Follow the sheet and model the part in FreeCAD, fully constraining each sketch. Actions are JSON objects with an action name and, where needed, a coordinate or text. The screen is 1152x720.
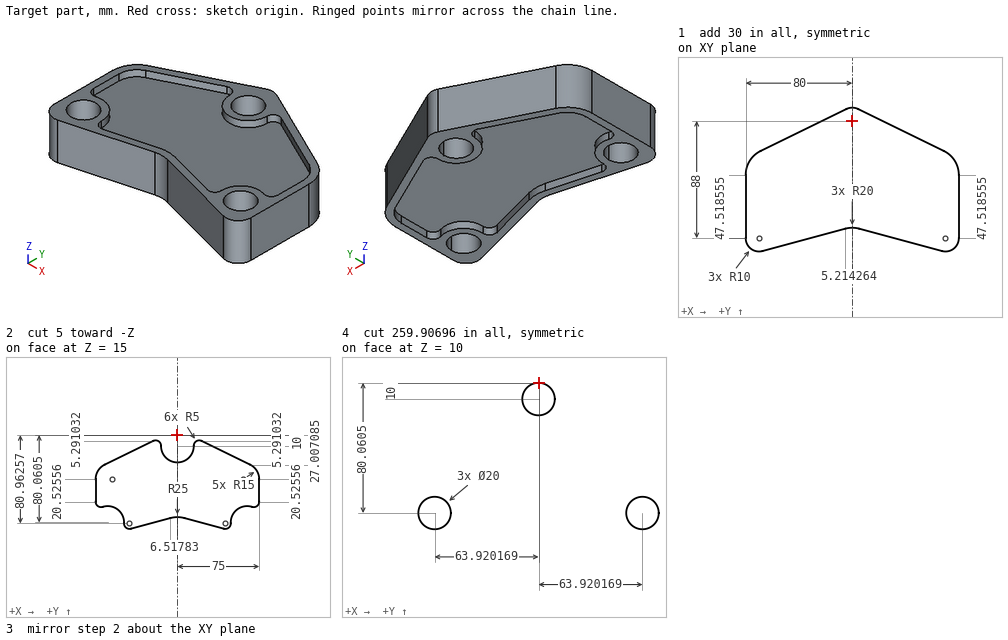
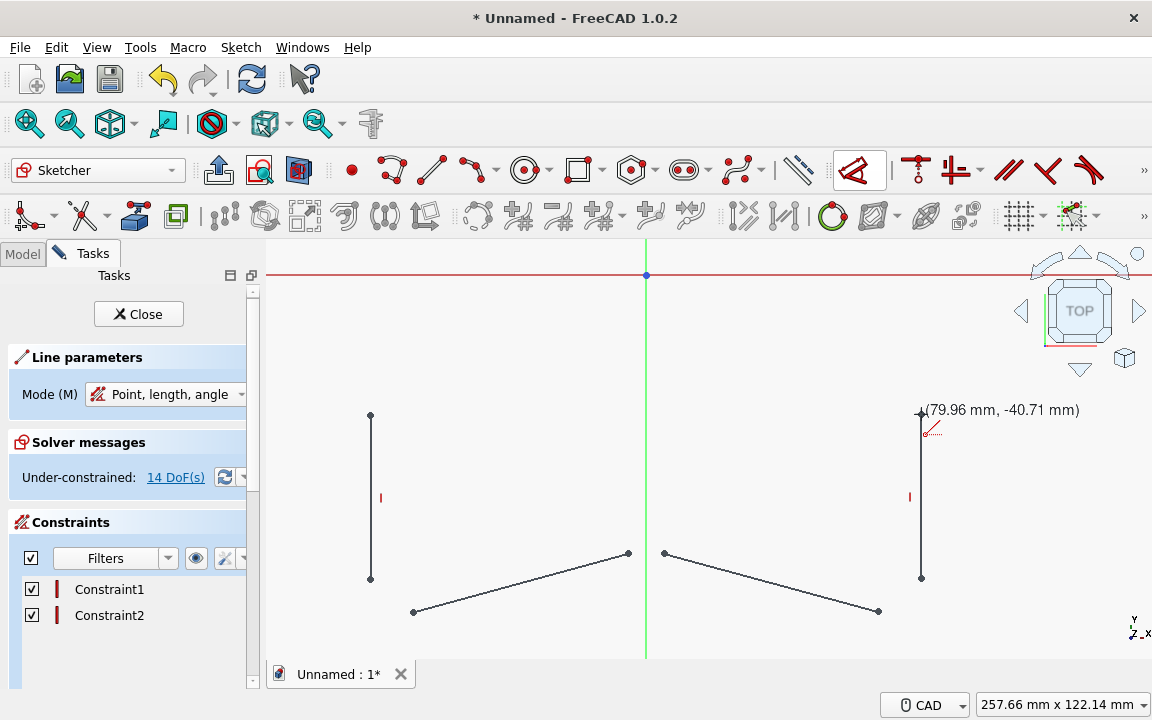
{"action": "left_click", "coordinate": [883, 352]}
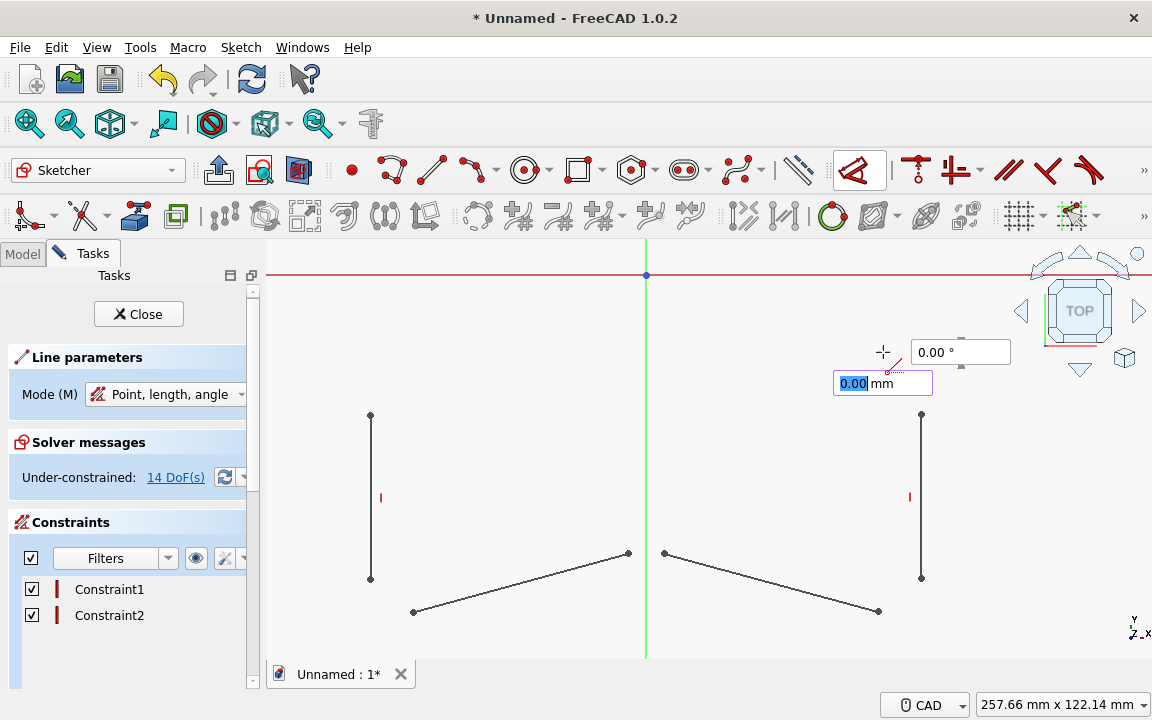
{"action": "scroll", "coordinate": [629, 496], "scroll_direction": "down", "scroll_amount": 2}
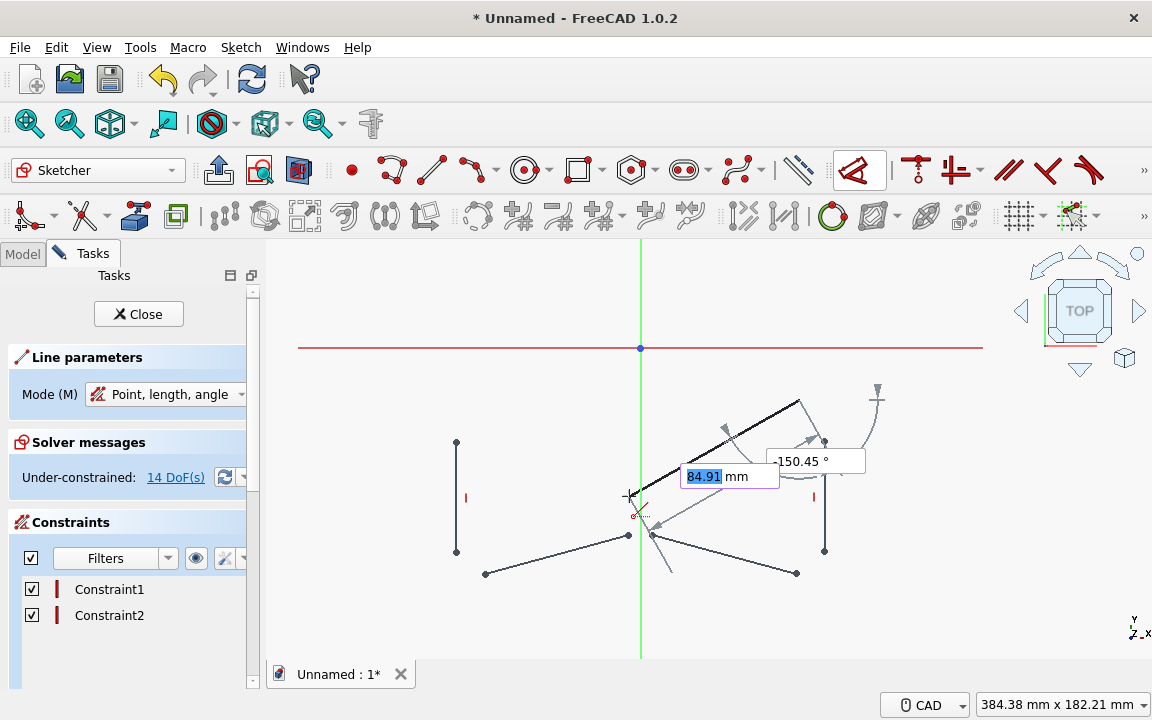
{"action": "scroll", "coordinate": [651, 327], "scroll_direction": "up", "scroll_amount": 3}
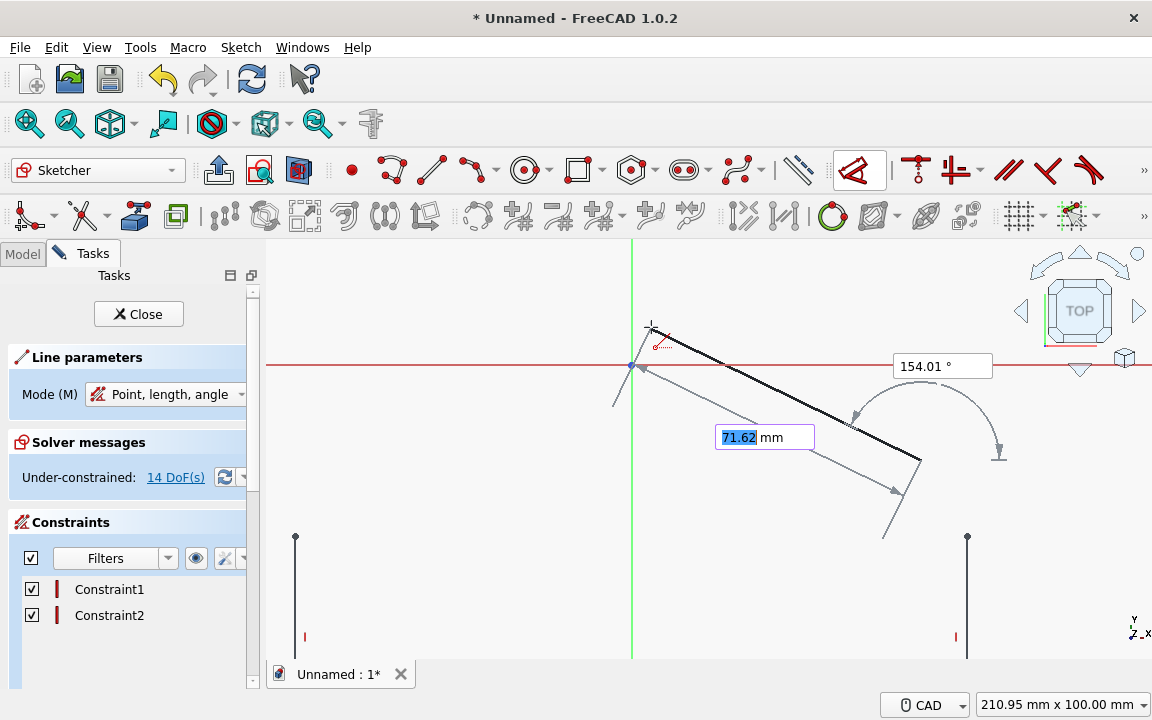
{"action": "left_click", "coordinate": [650, 328]}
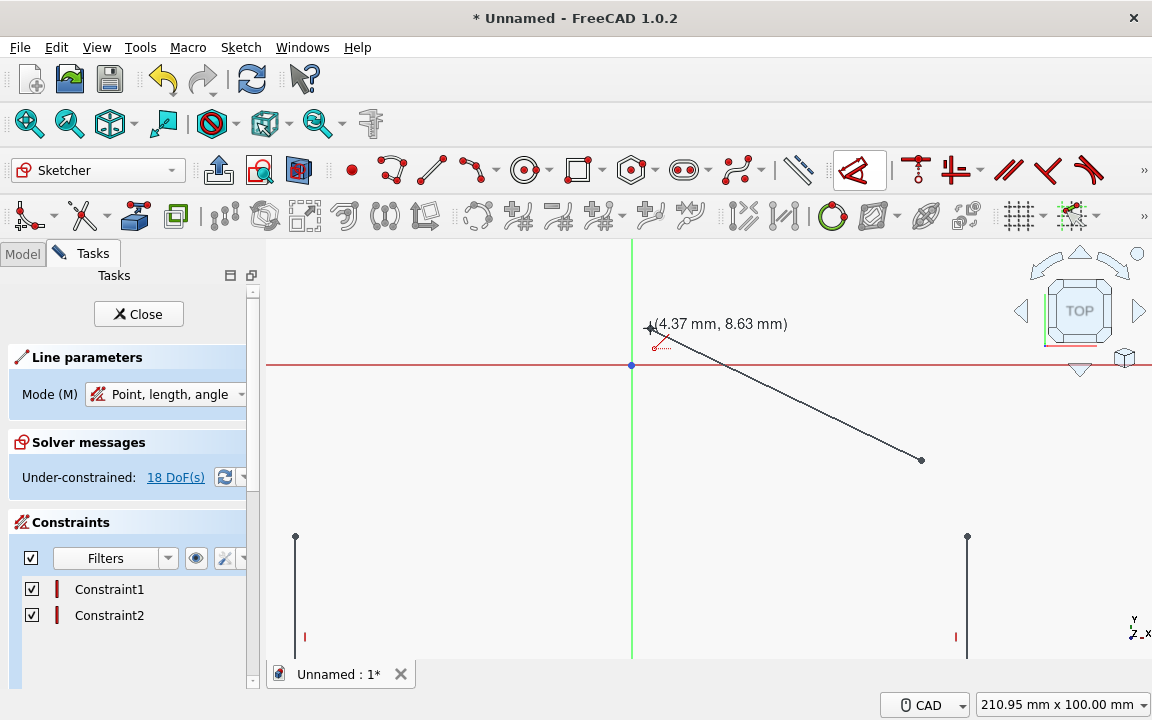
{"action": "left_click", "coordinate": [613, 328]}
{"action": "left_click", "coordinate": [343, 460]}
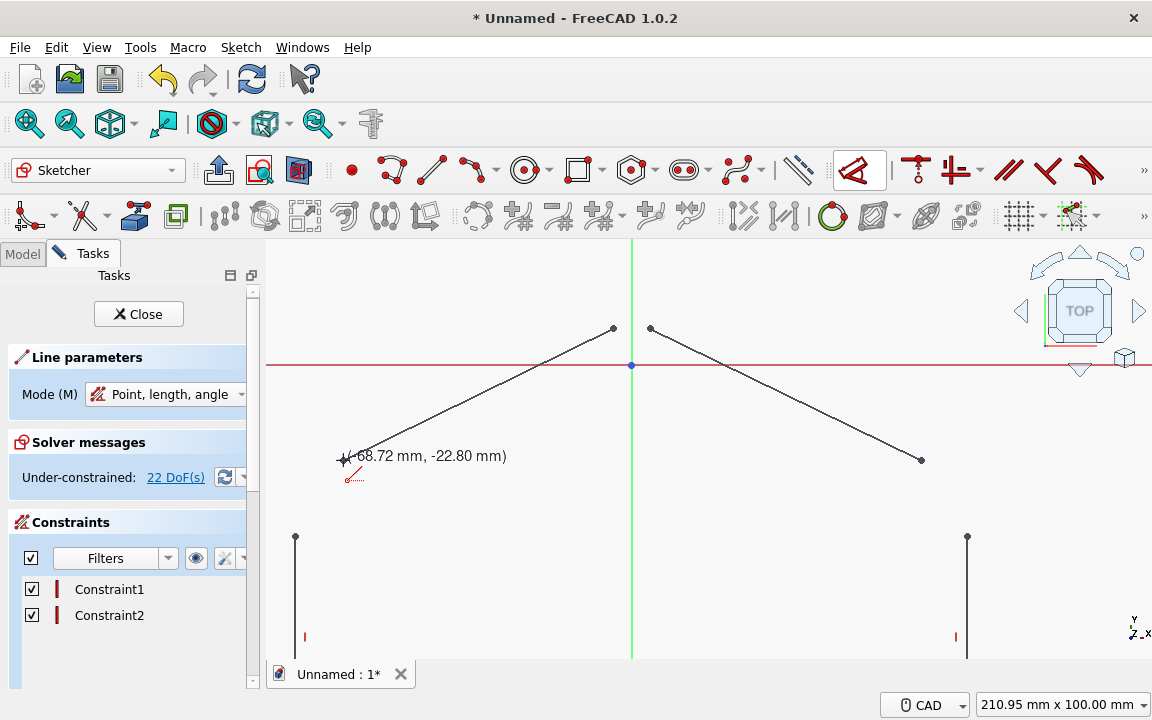
{"action": "left_click", "coordinate": [472, 170]}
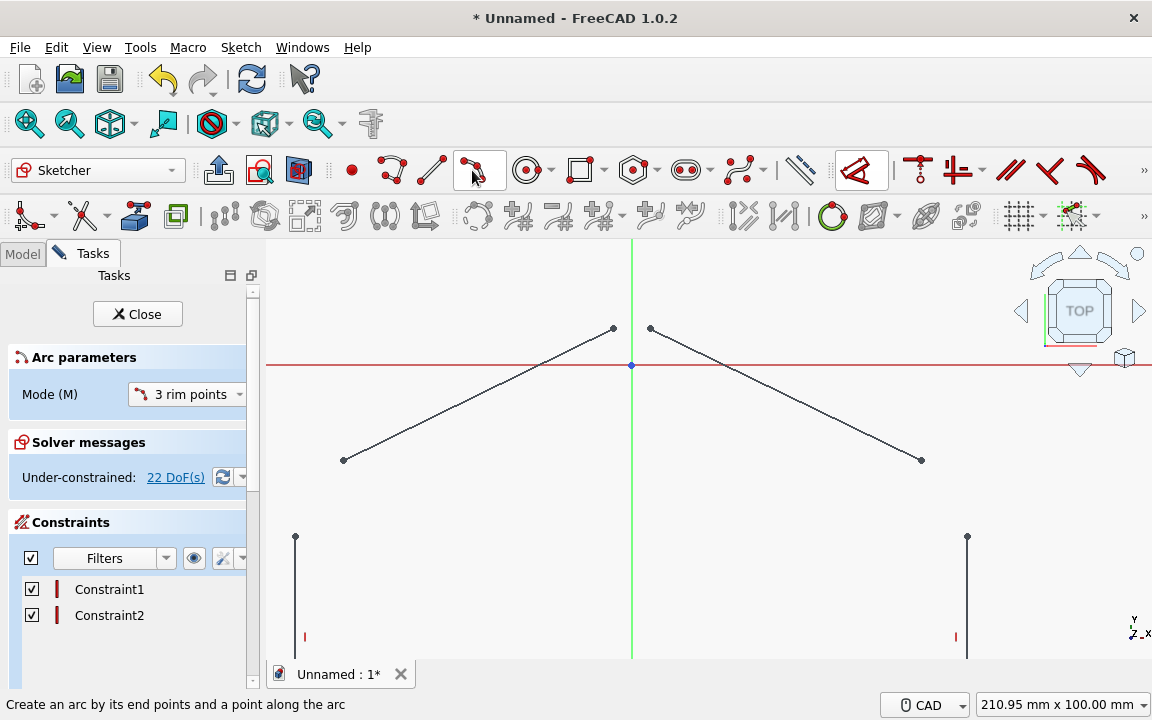
{"action": "scroll", "coordinate": [651, 327], "scroll_direction": "down", "scroll_amount": 3}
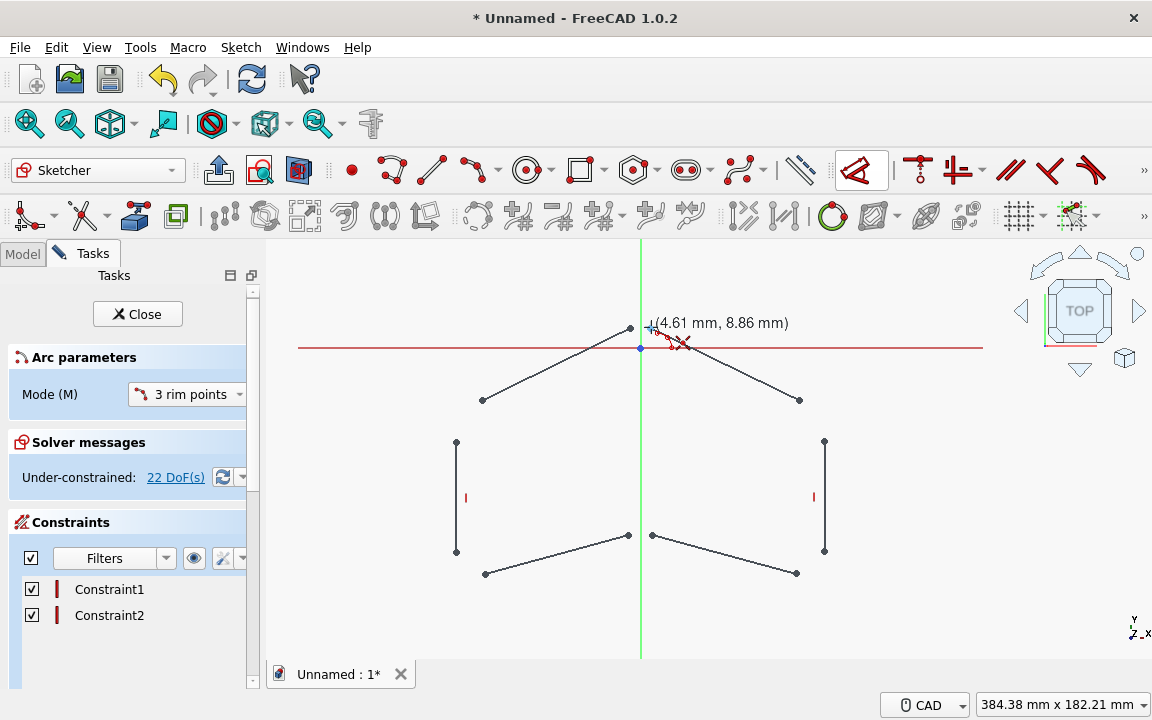
{"action": "left_click", "coordinate": [456, 552]}
{"action": "left_click", "coordinate": [485, 574]}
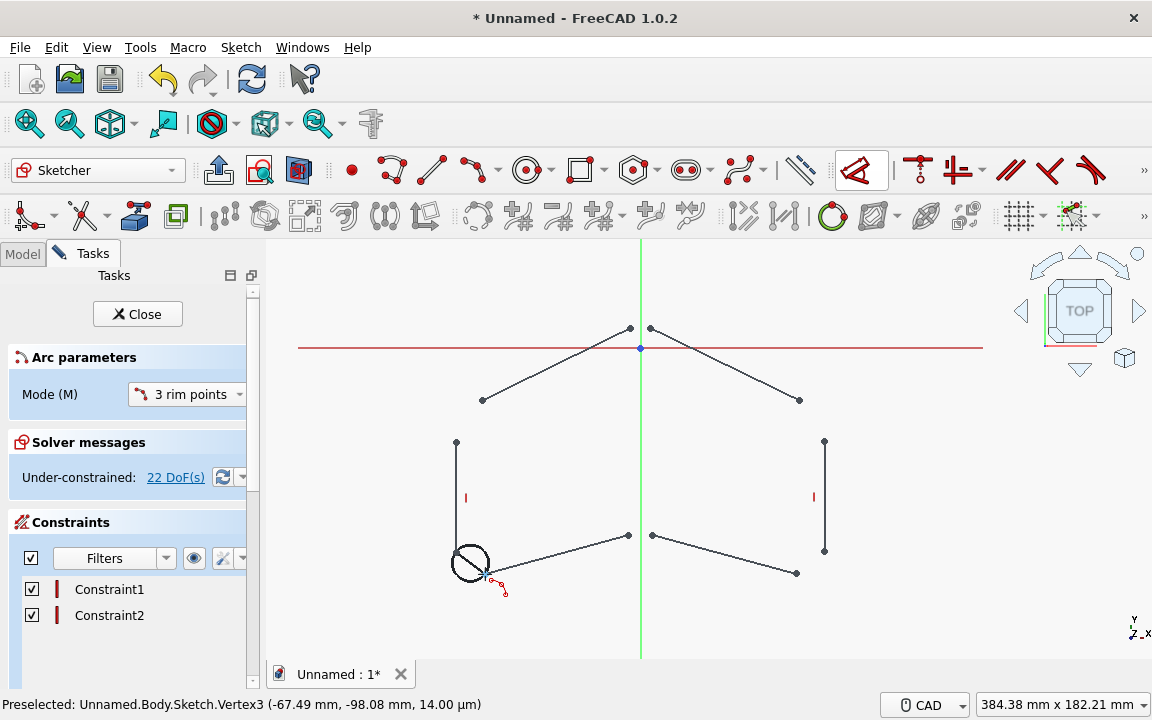
{"action": "scroll", "coordinate": [465, 569], "scroll_direction": "up", "scroll_amount": 3}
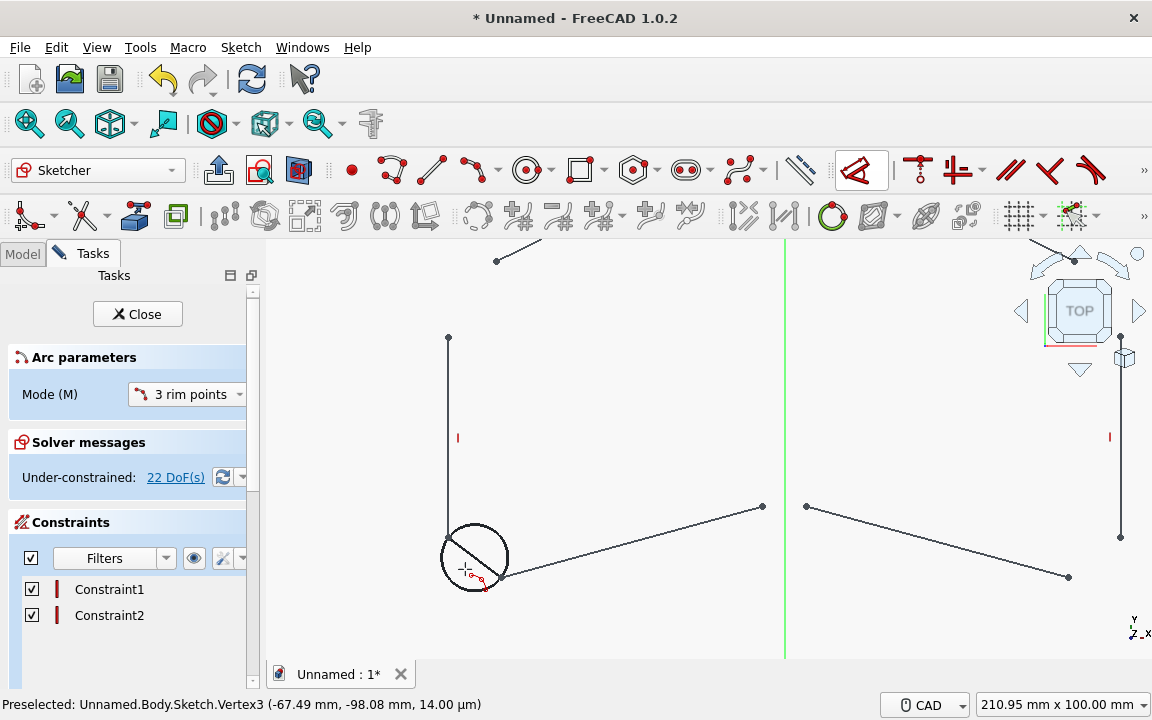
{"action": "left_click", "coordinate": [465, 569]}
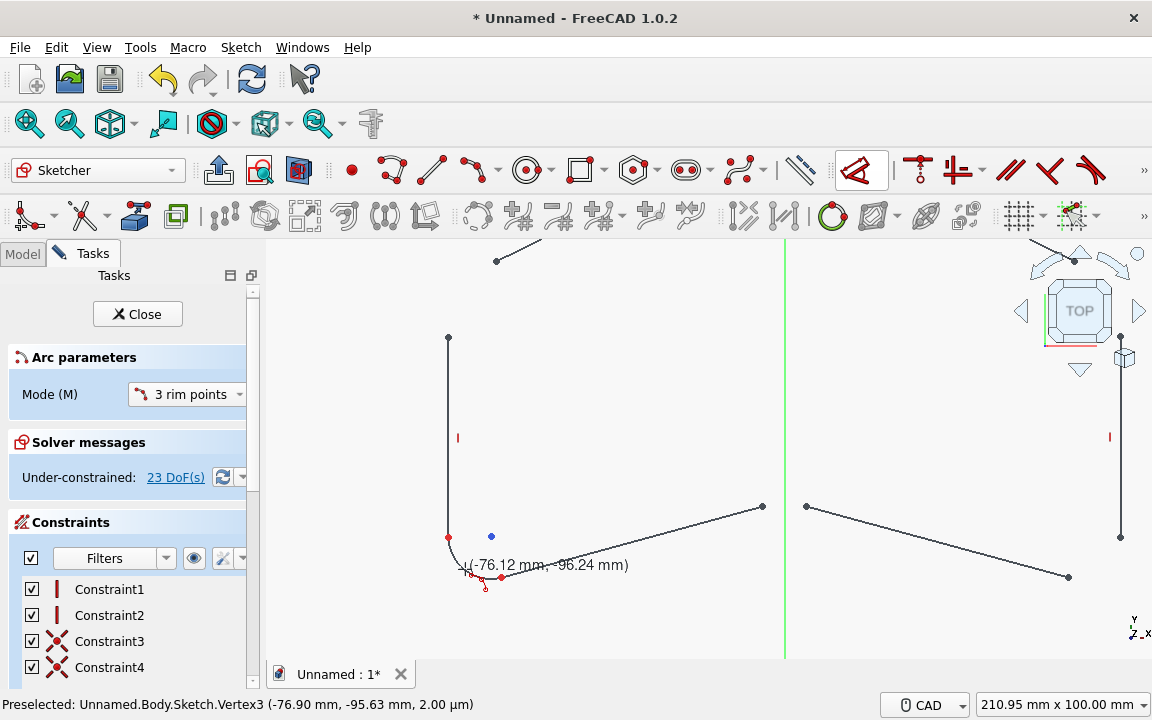
{"action": "left_click", "coordinate": [763, 507]}
{"action": "left_click", "coordinate": [807, 507]}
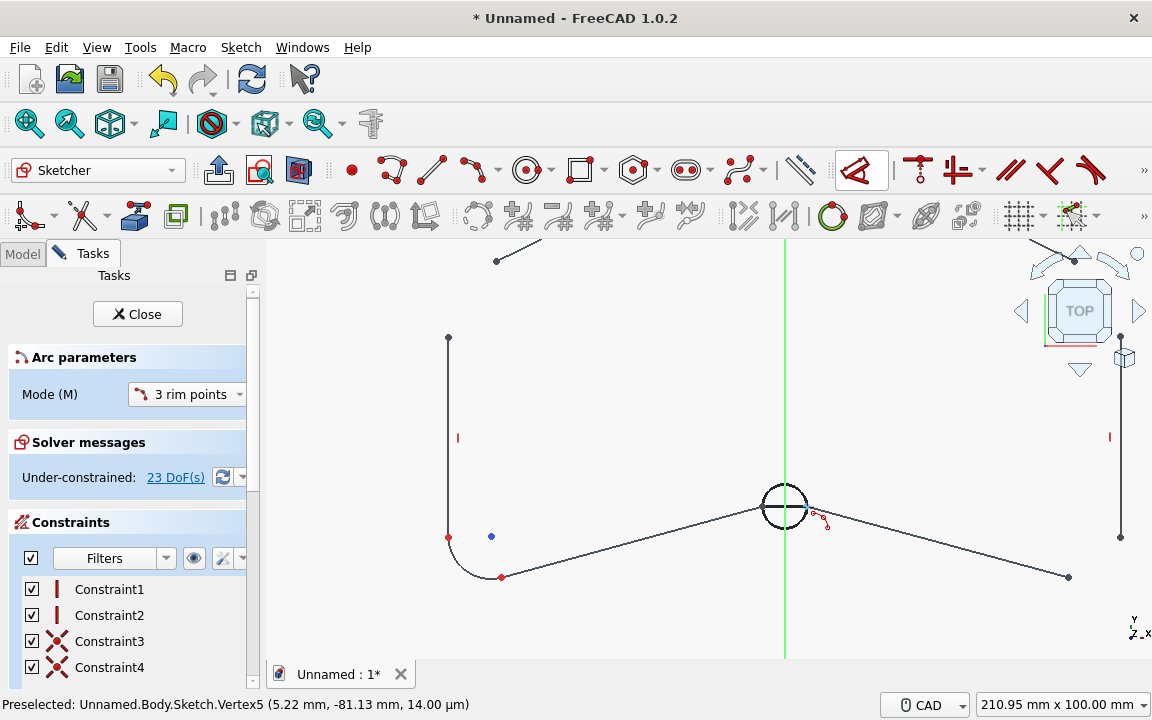
{"action": "scroll", "coordinate": [789, 503], "scroll_direction": "up", "scroll_amount": 9}